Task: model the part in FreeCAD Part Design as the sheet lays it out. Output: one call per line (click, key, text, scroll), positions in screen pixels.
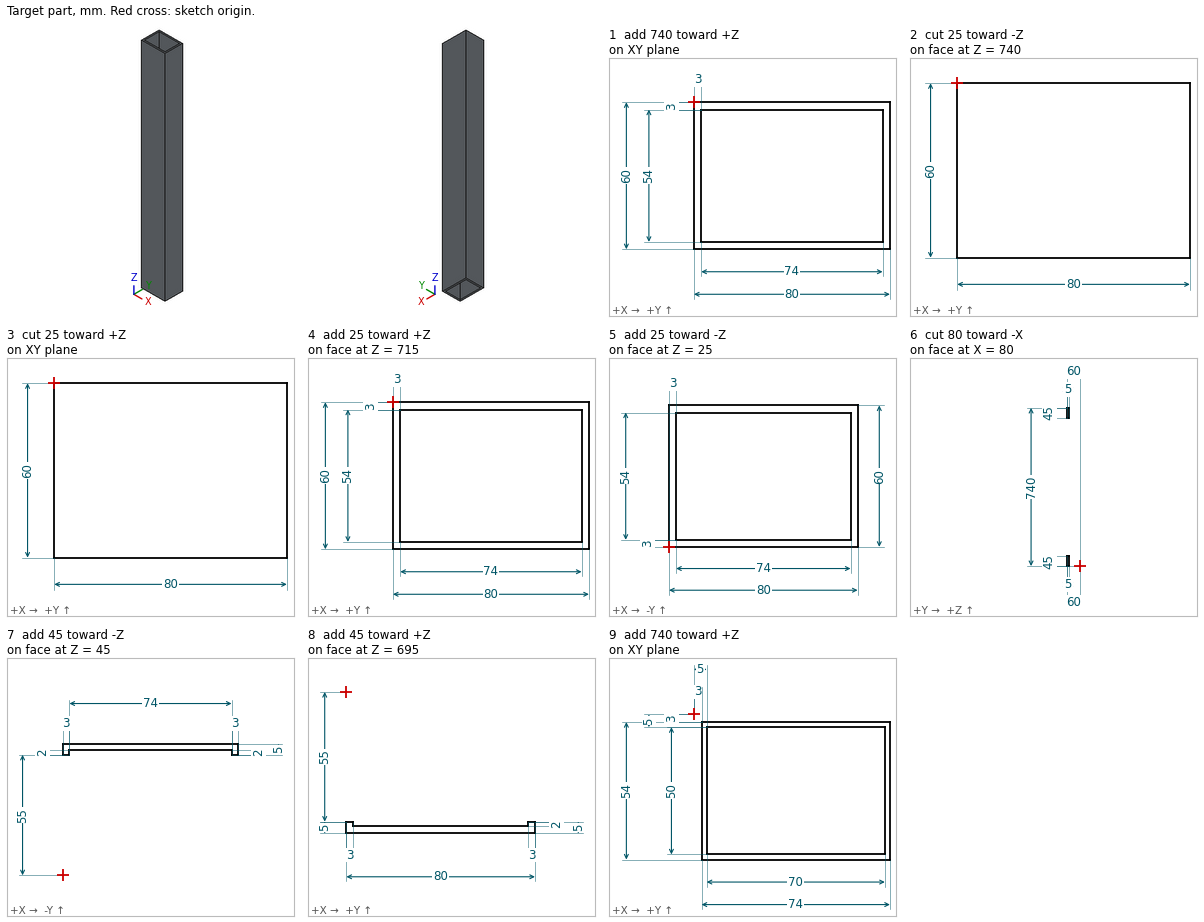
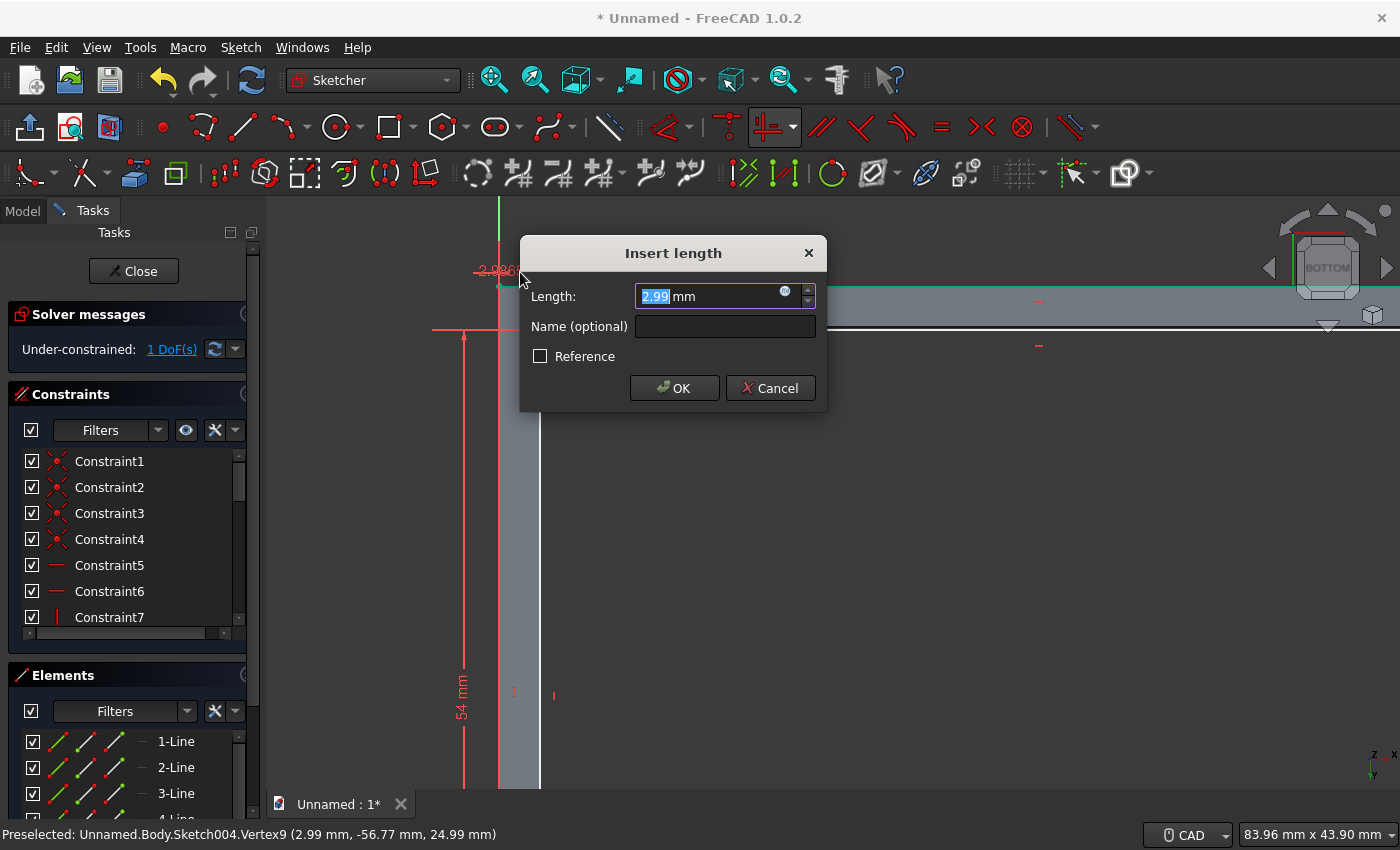
text(3)
key(Return)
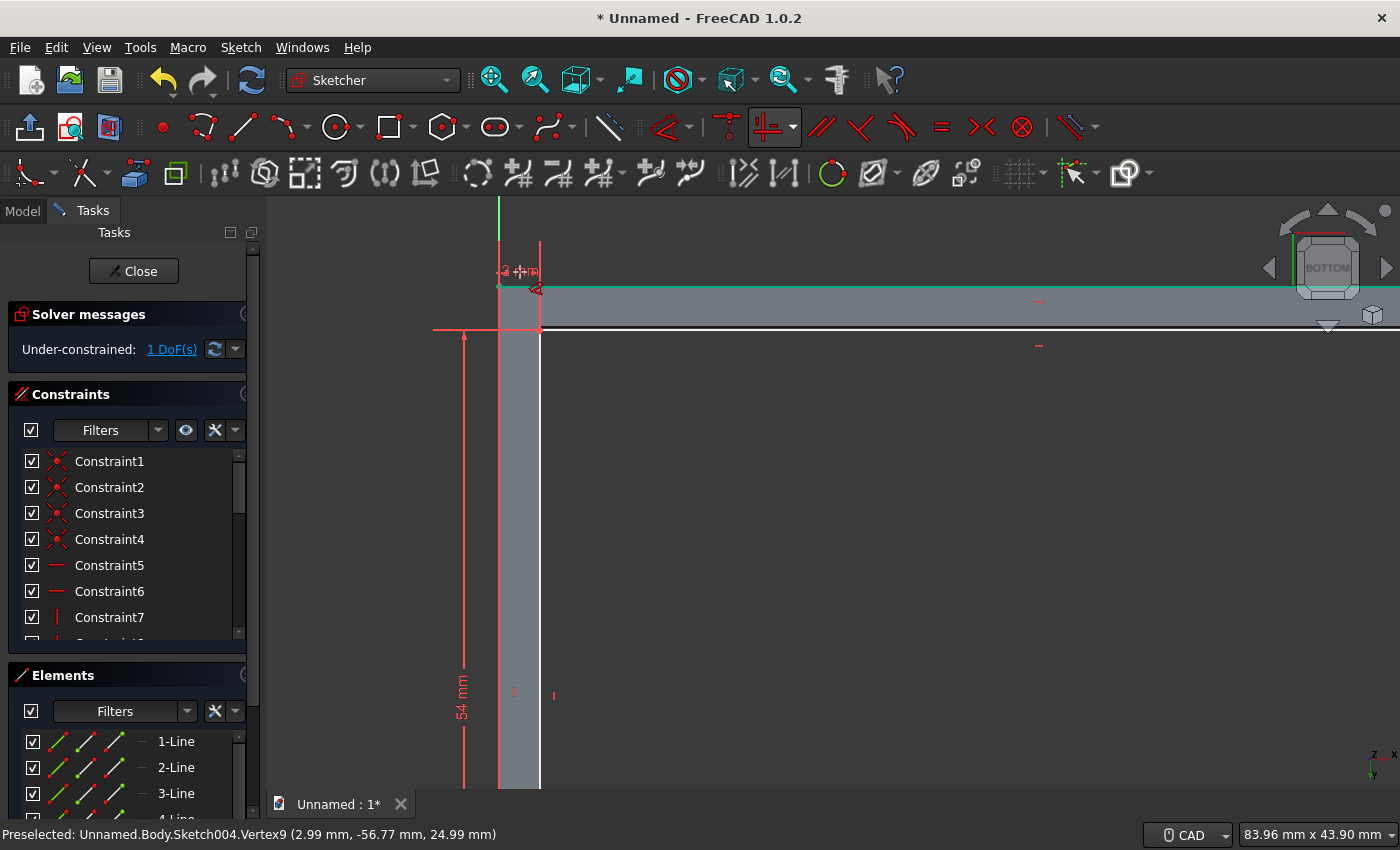
scroll(540, 330, down, 4)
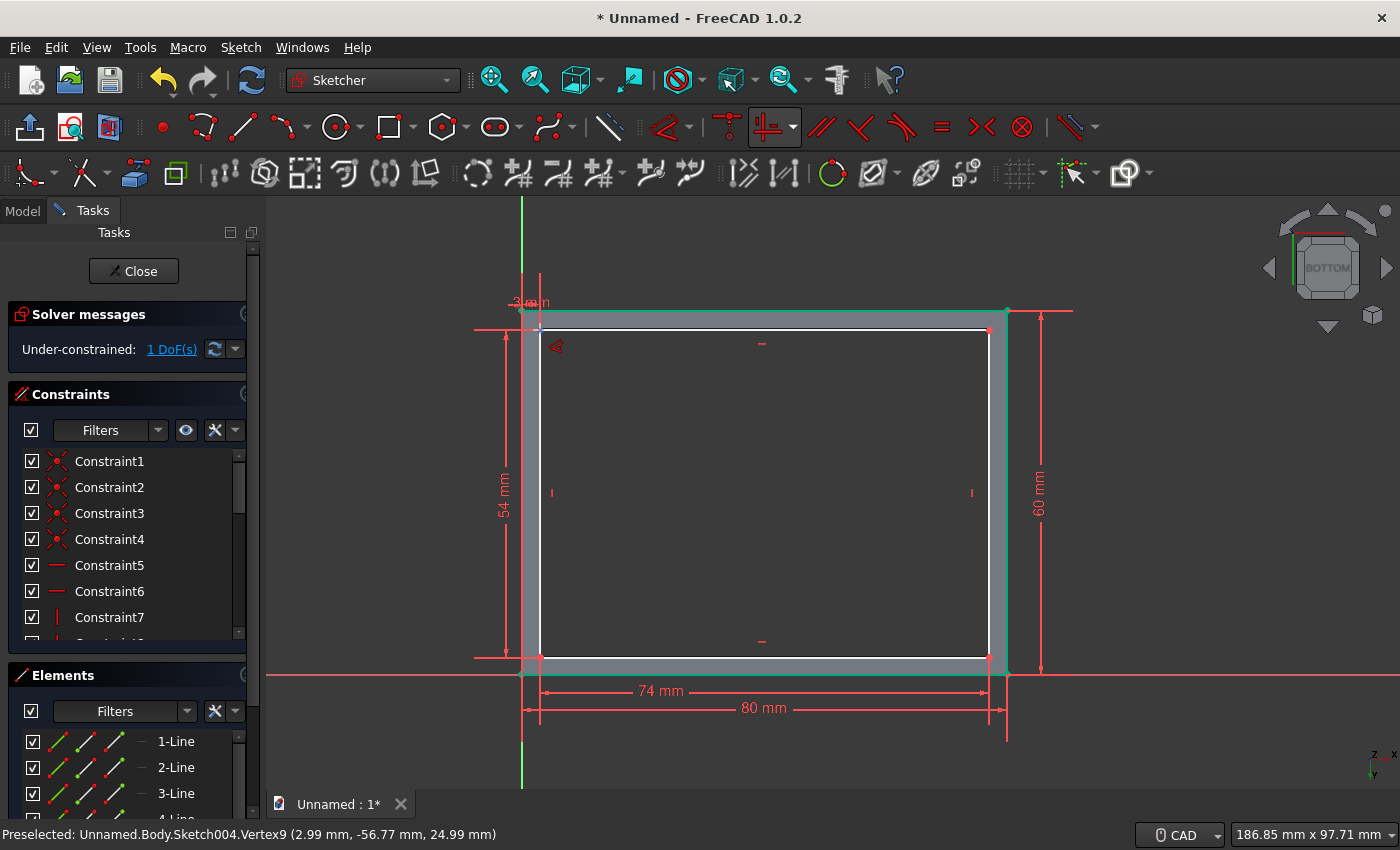
scroll(540, 658, up, 4)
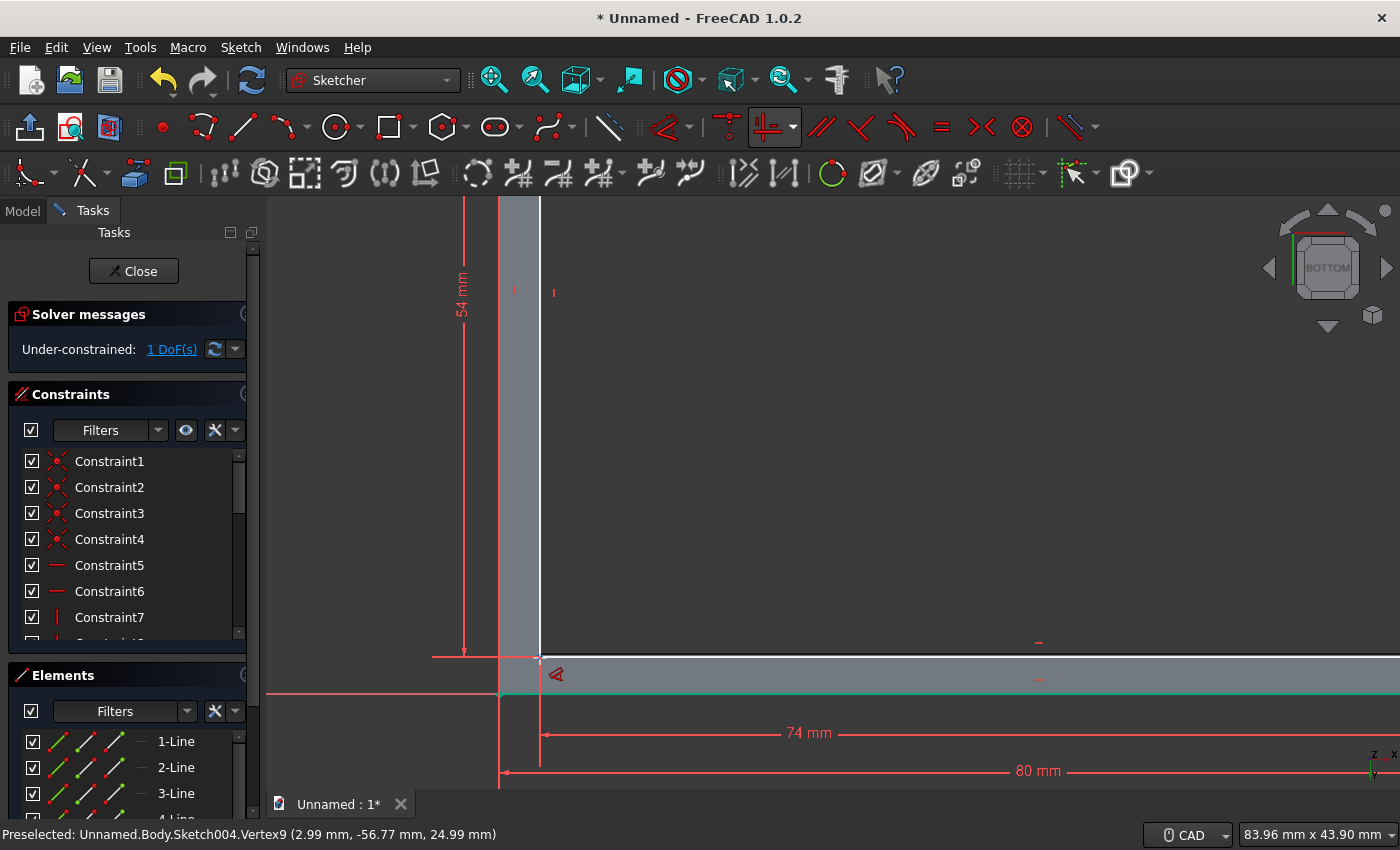
click(540, 657)
click(465, 676)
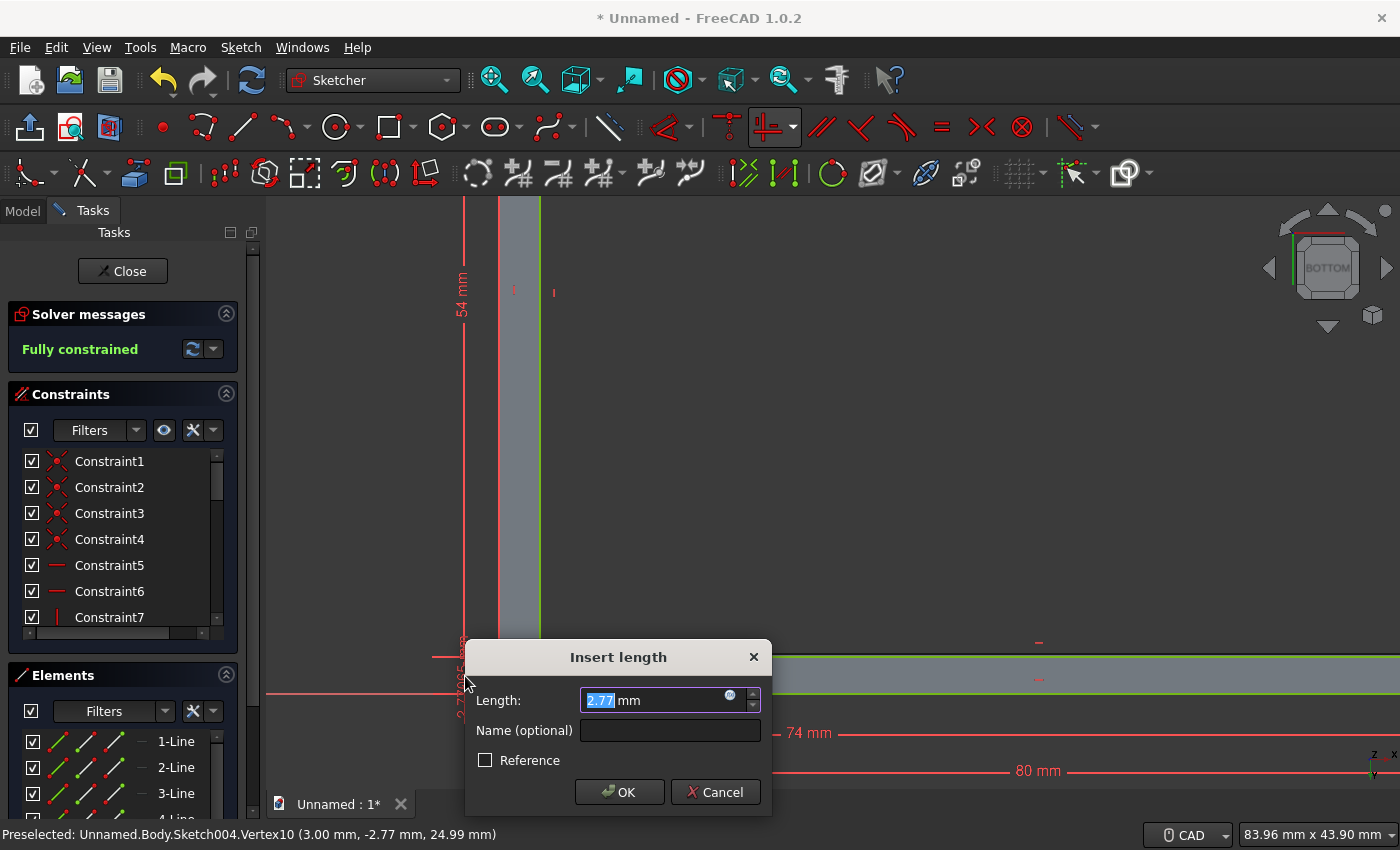
text(3)
key(Return)
key(Escape)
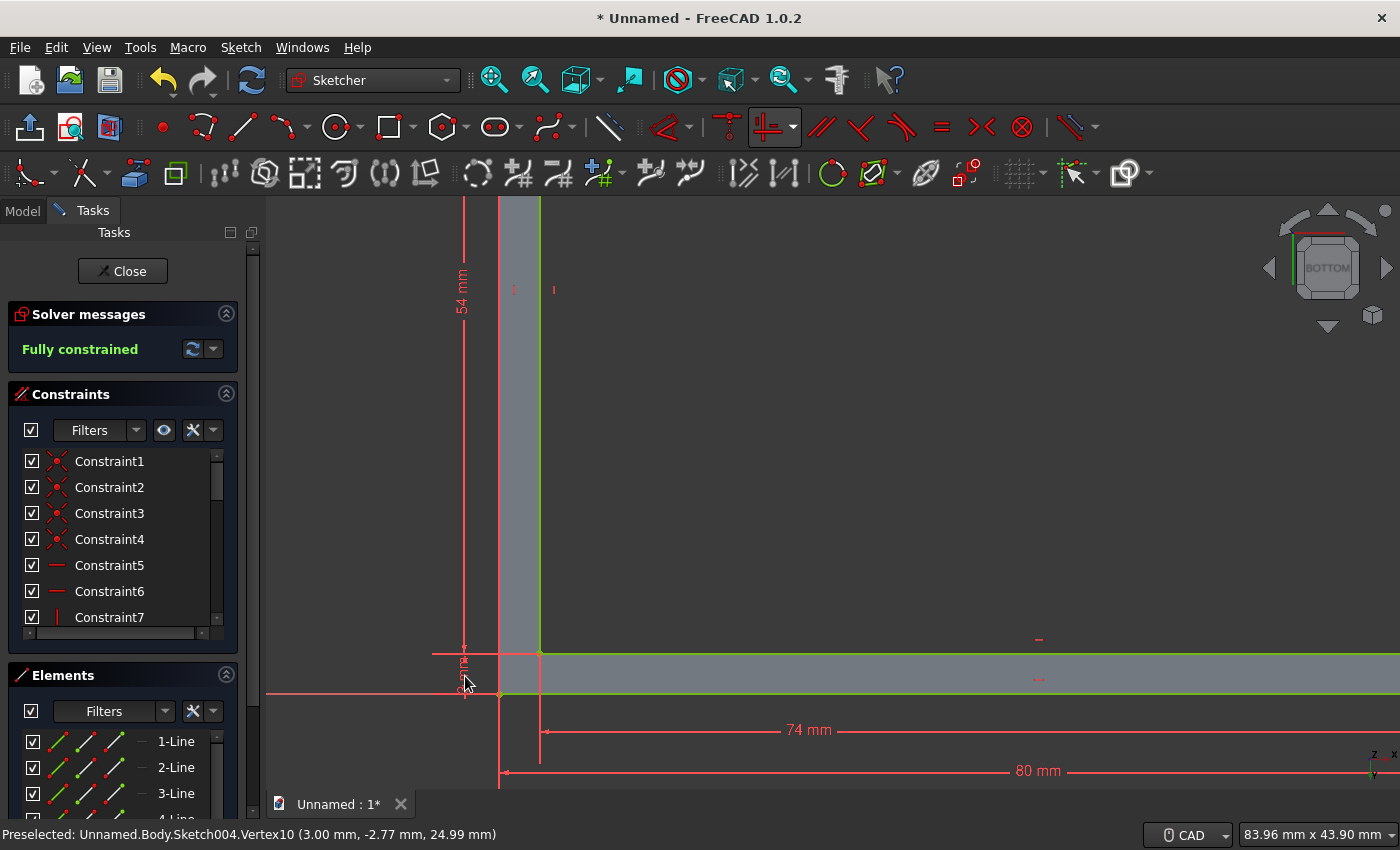
click(123, 271)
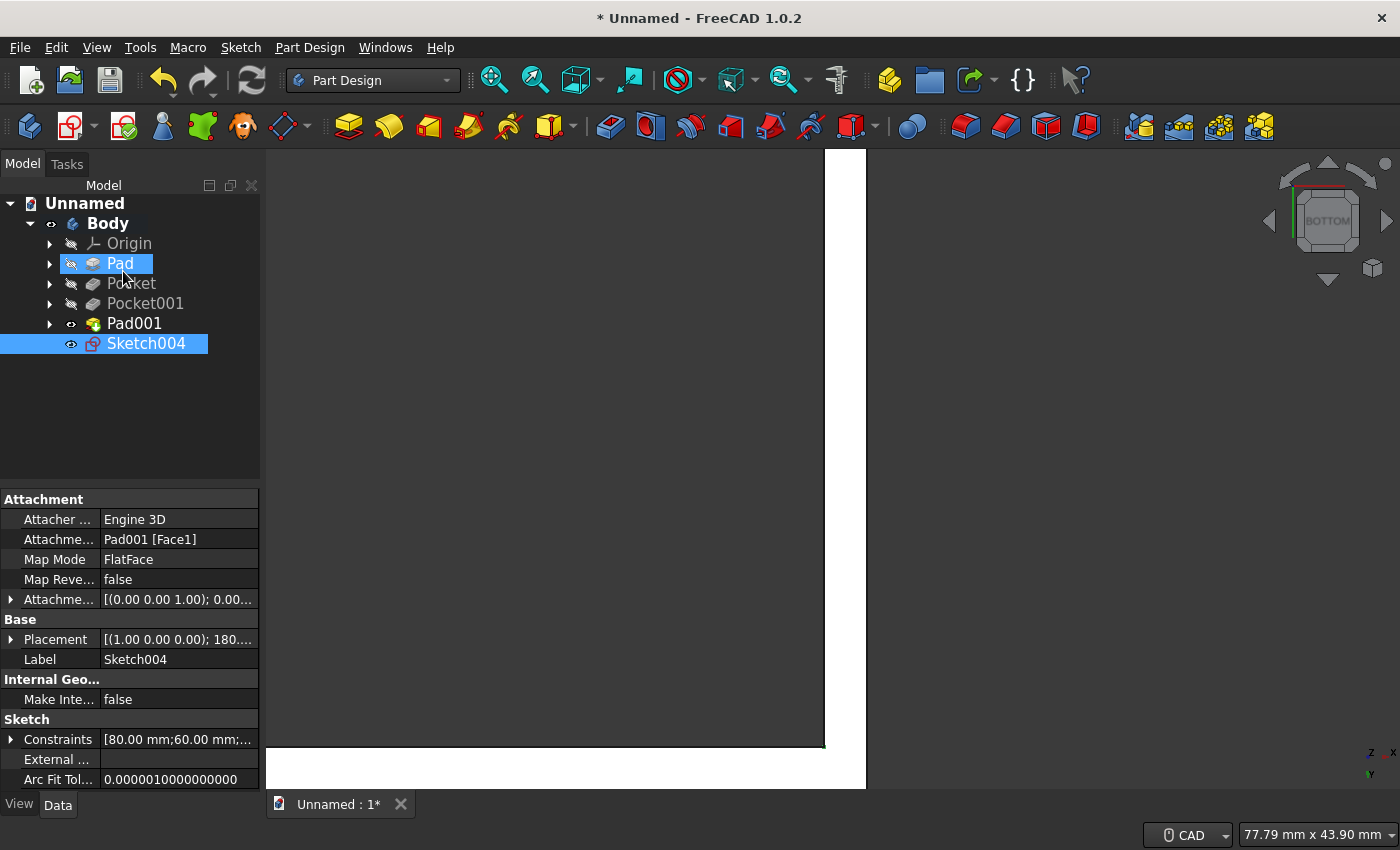
click(350, 126)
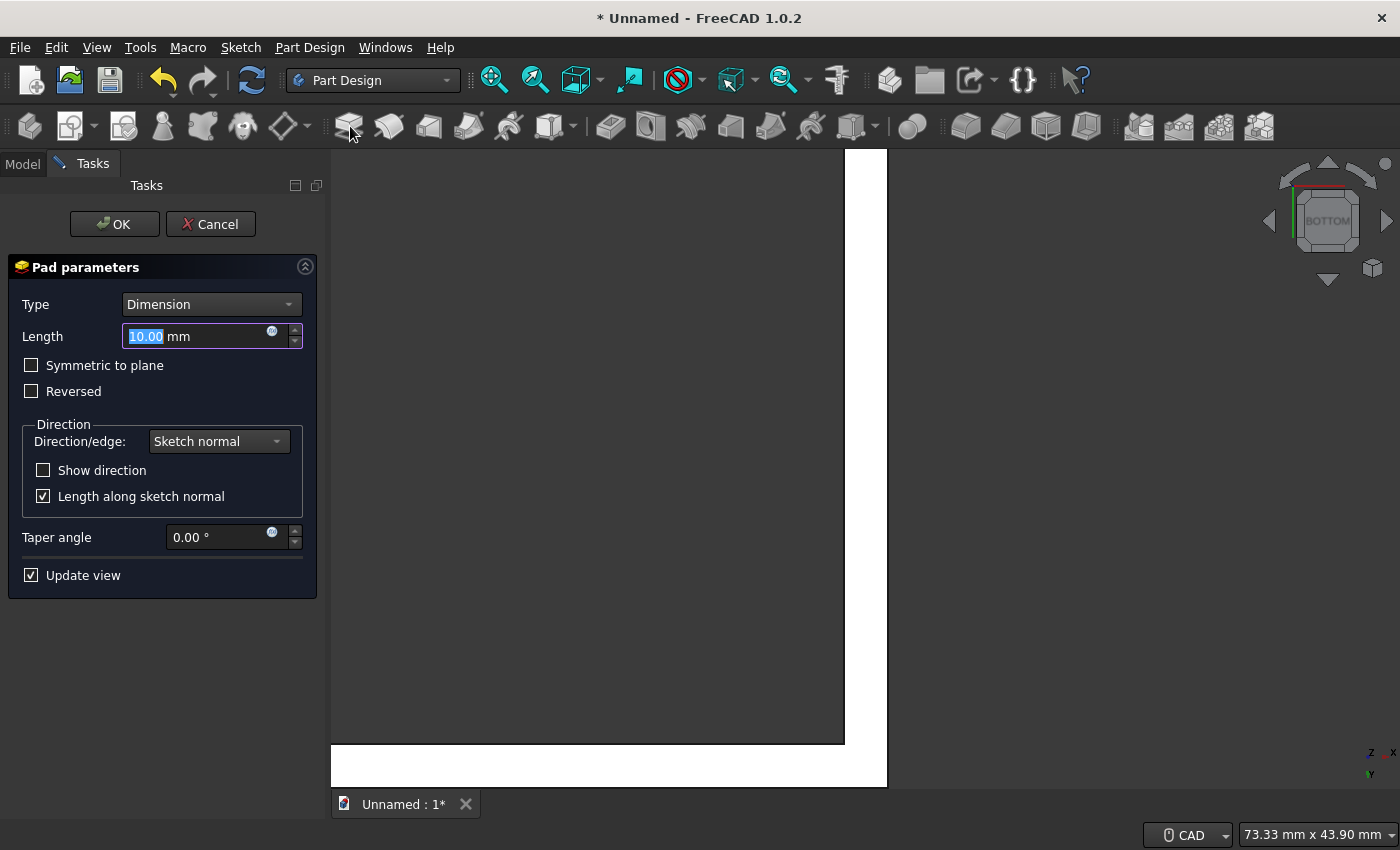
text(25)
key(Tab)